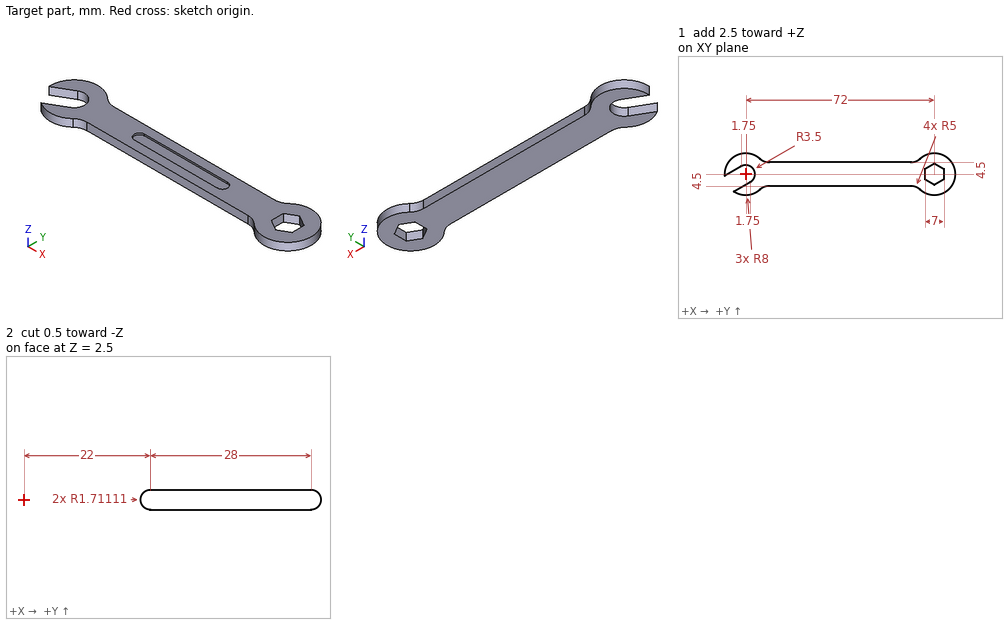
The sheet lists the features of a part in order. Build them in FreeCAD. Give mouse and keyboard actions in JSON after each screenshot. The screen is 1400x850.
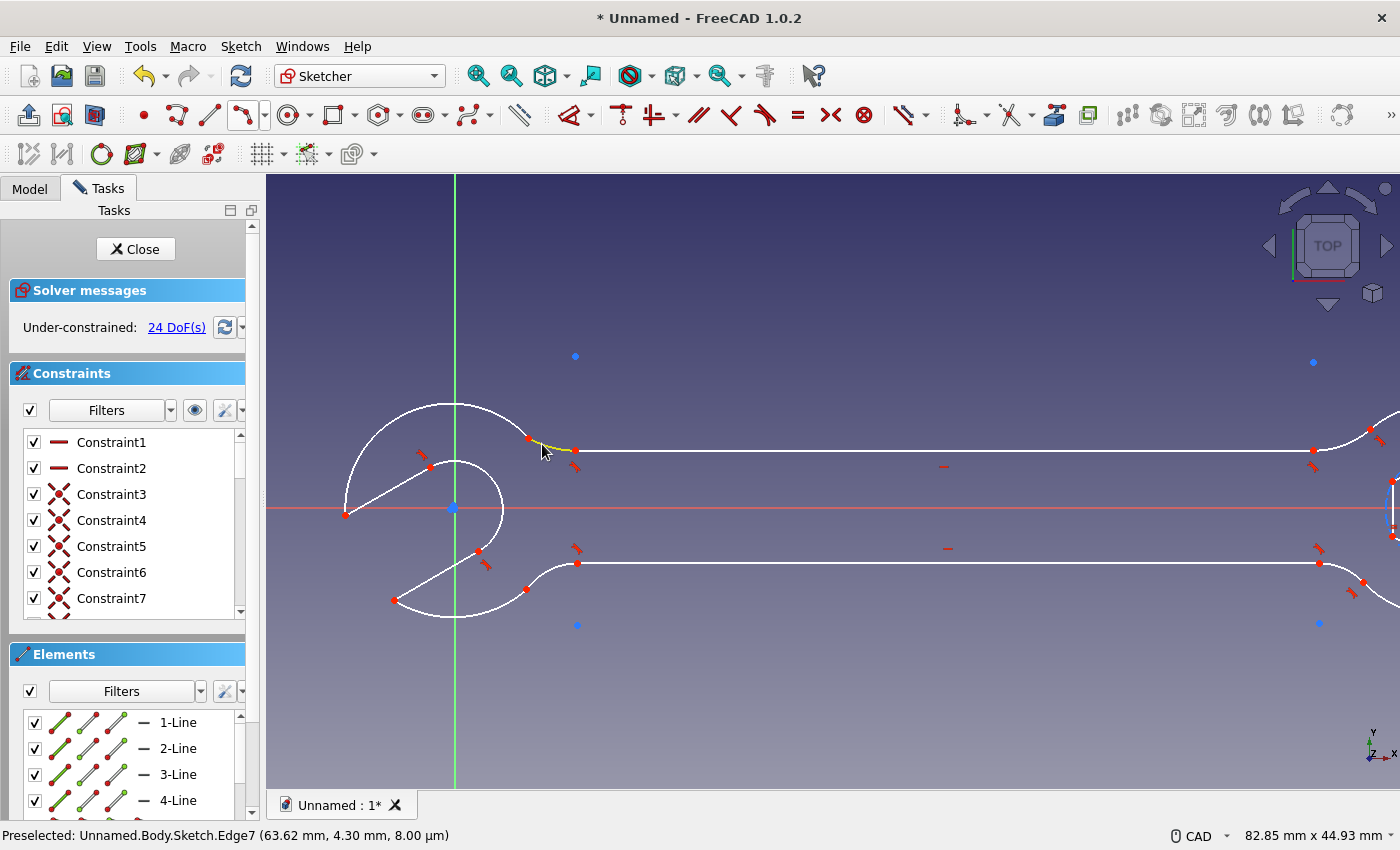
{"action": "left_click", "coordinate": [542, 444]}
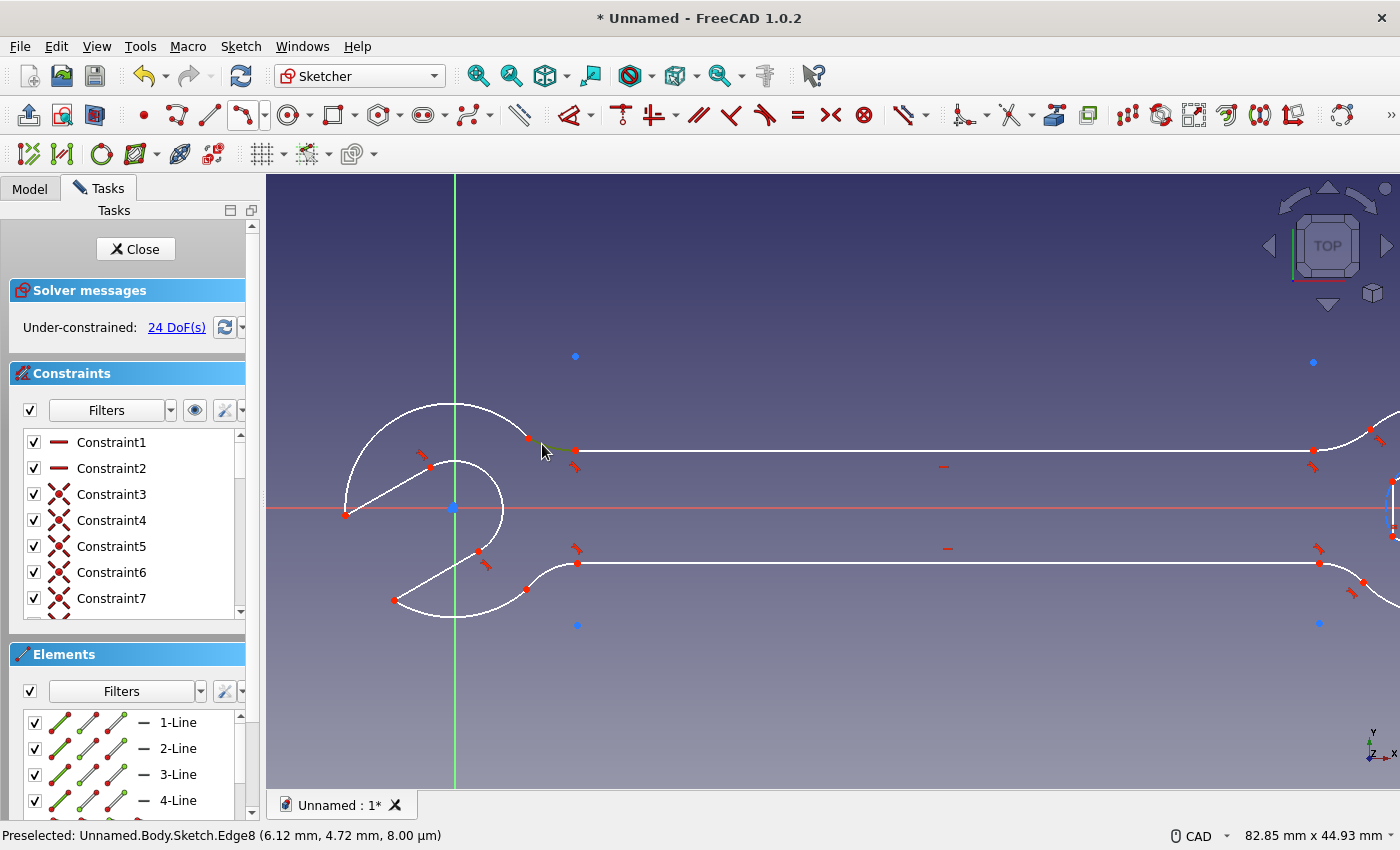
{"action": "left_click", "coordinate": [368, 443]}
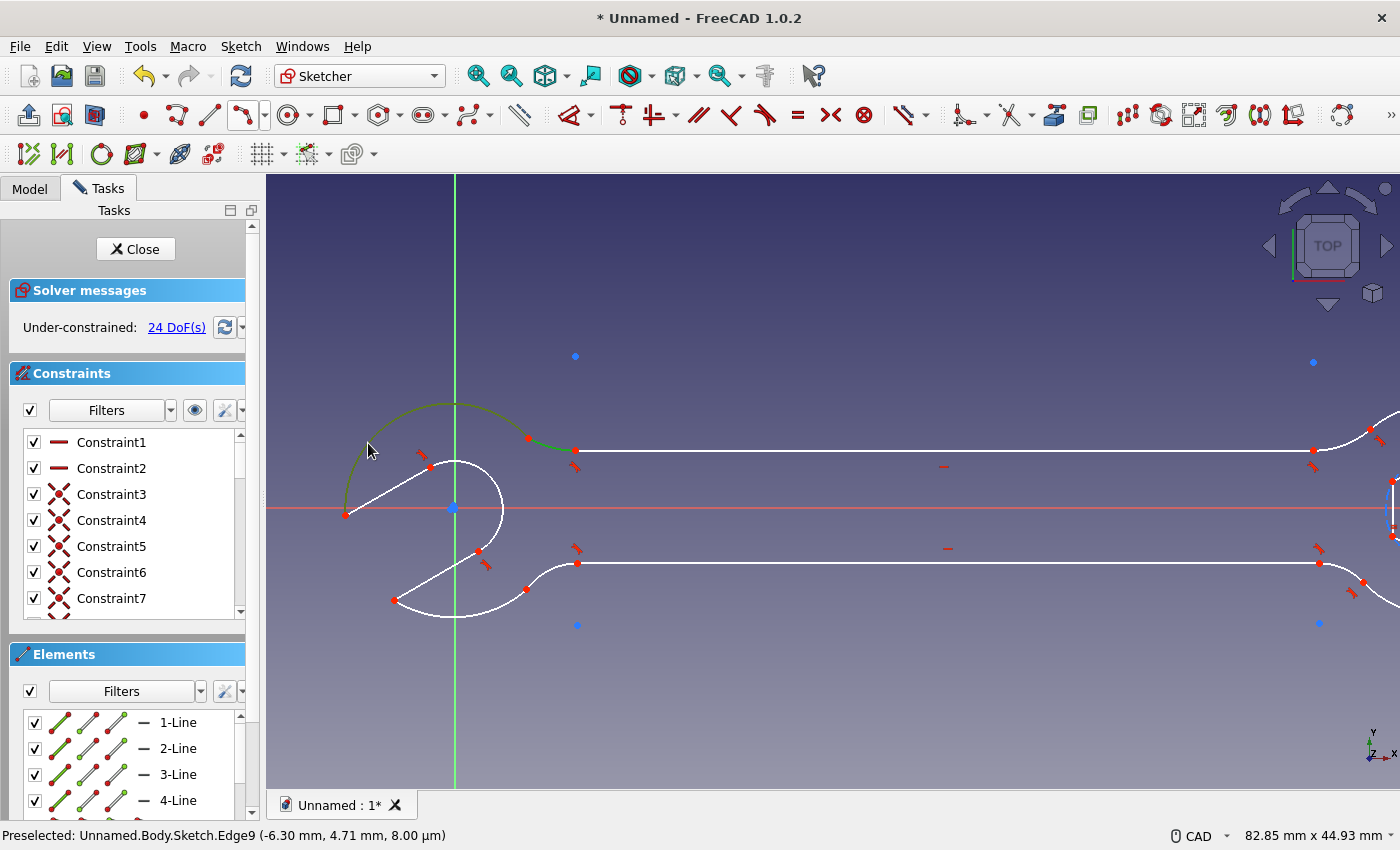
{"action": "key", "text": "t"}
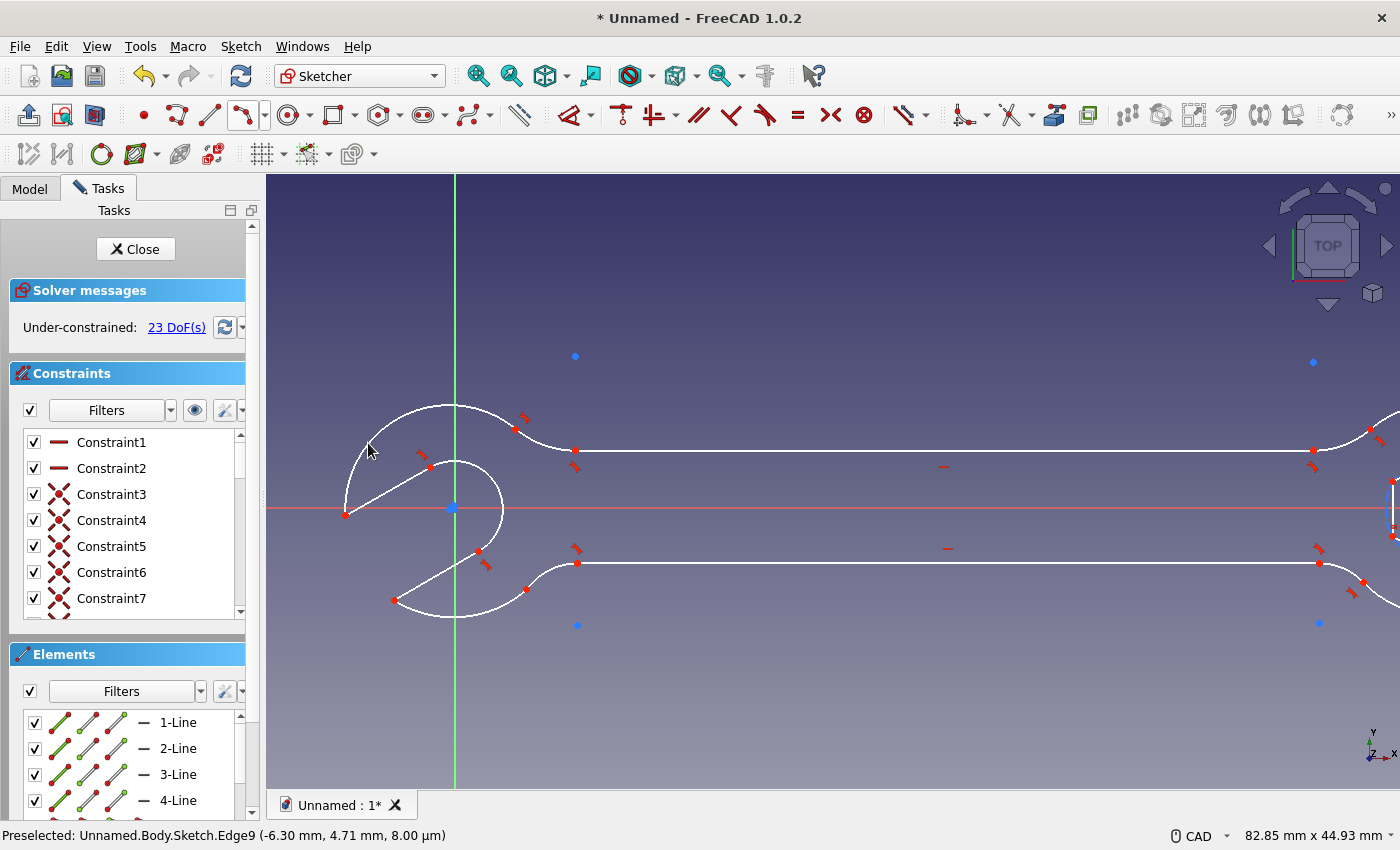
{"action": "left_click", "coordinate": [434, 616]}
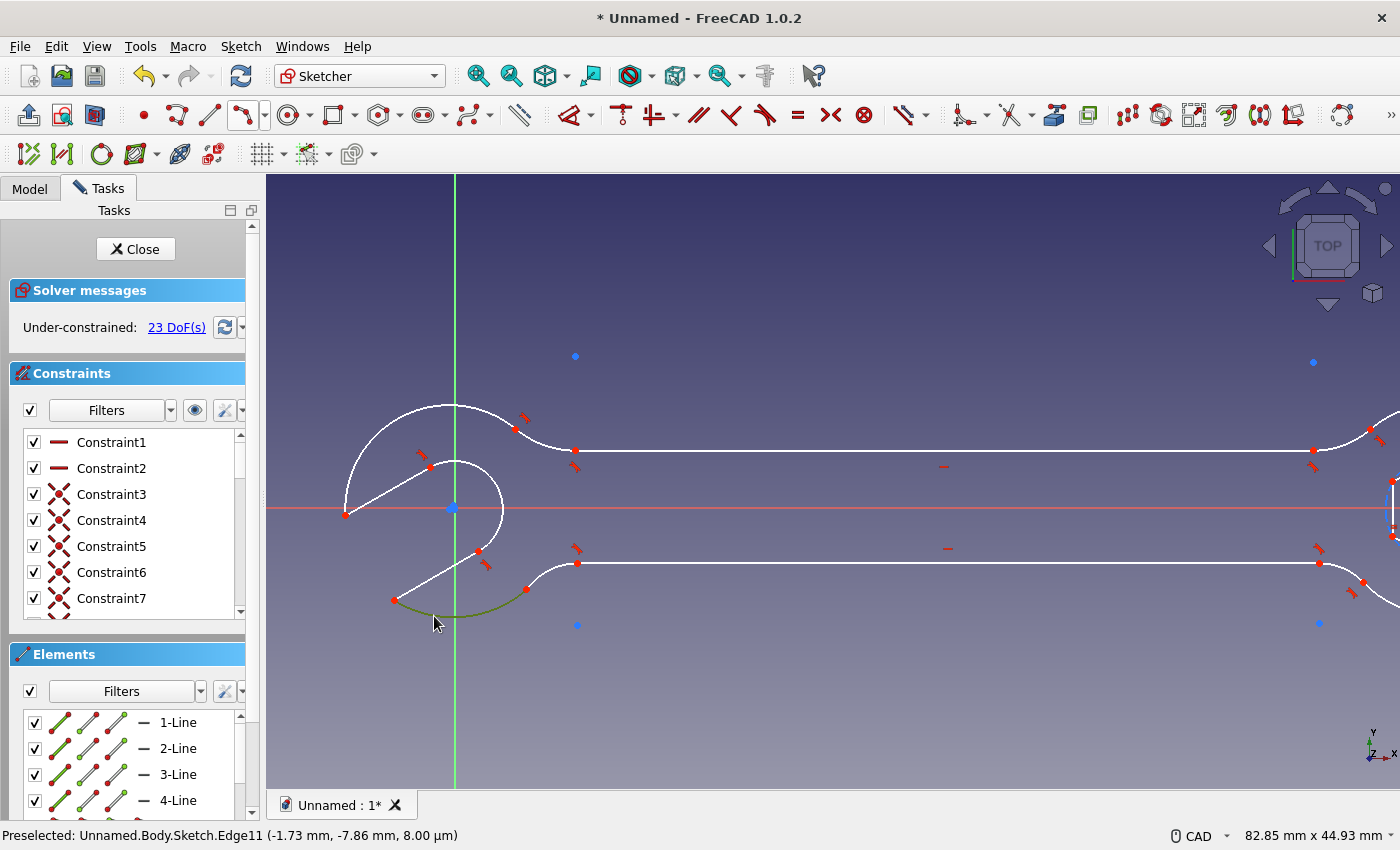
{"action": "left_click", "coordinate": [560, 566]}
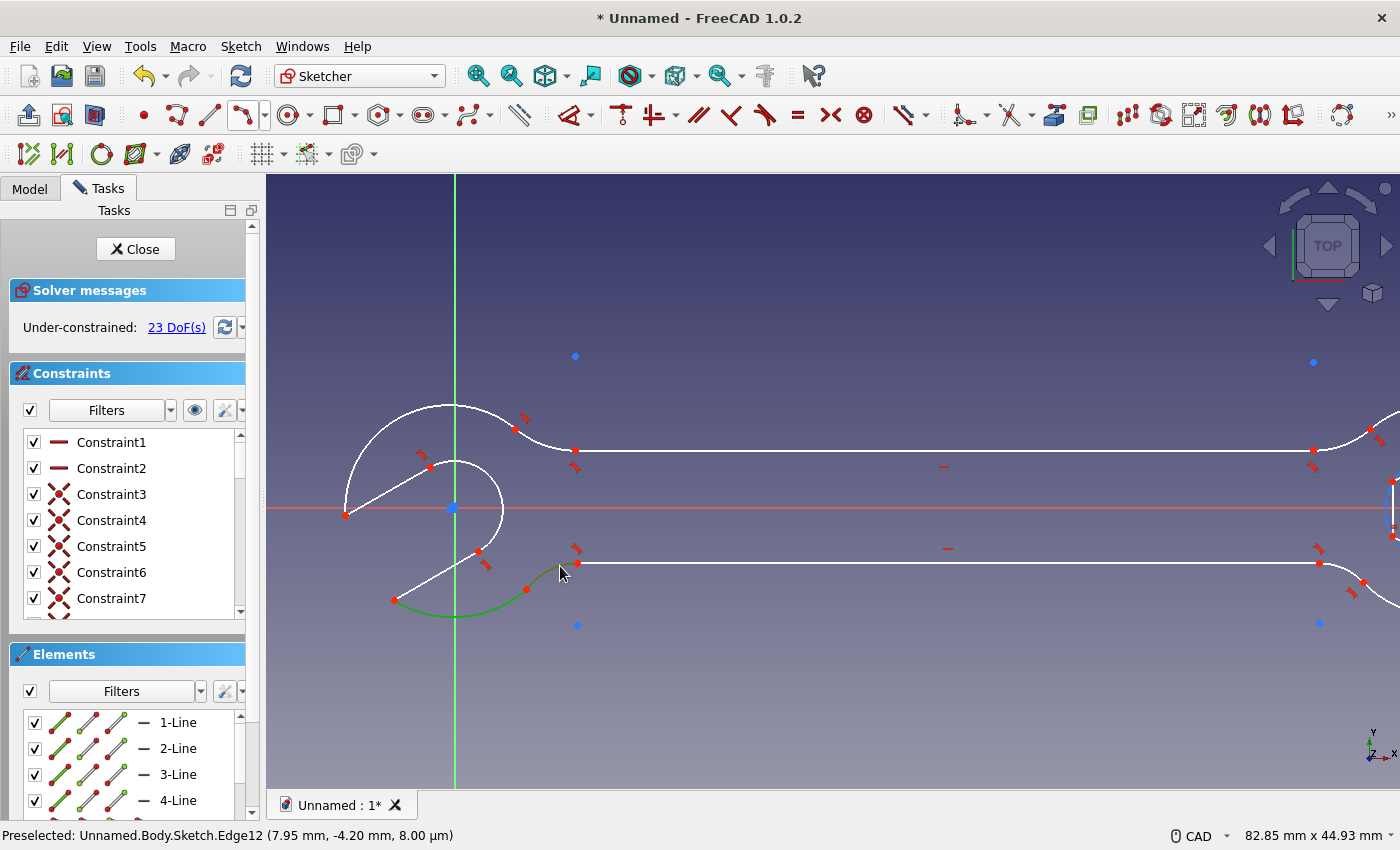
{"action": "left_click", "coordinate": [765, 116]}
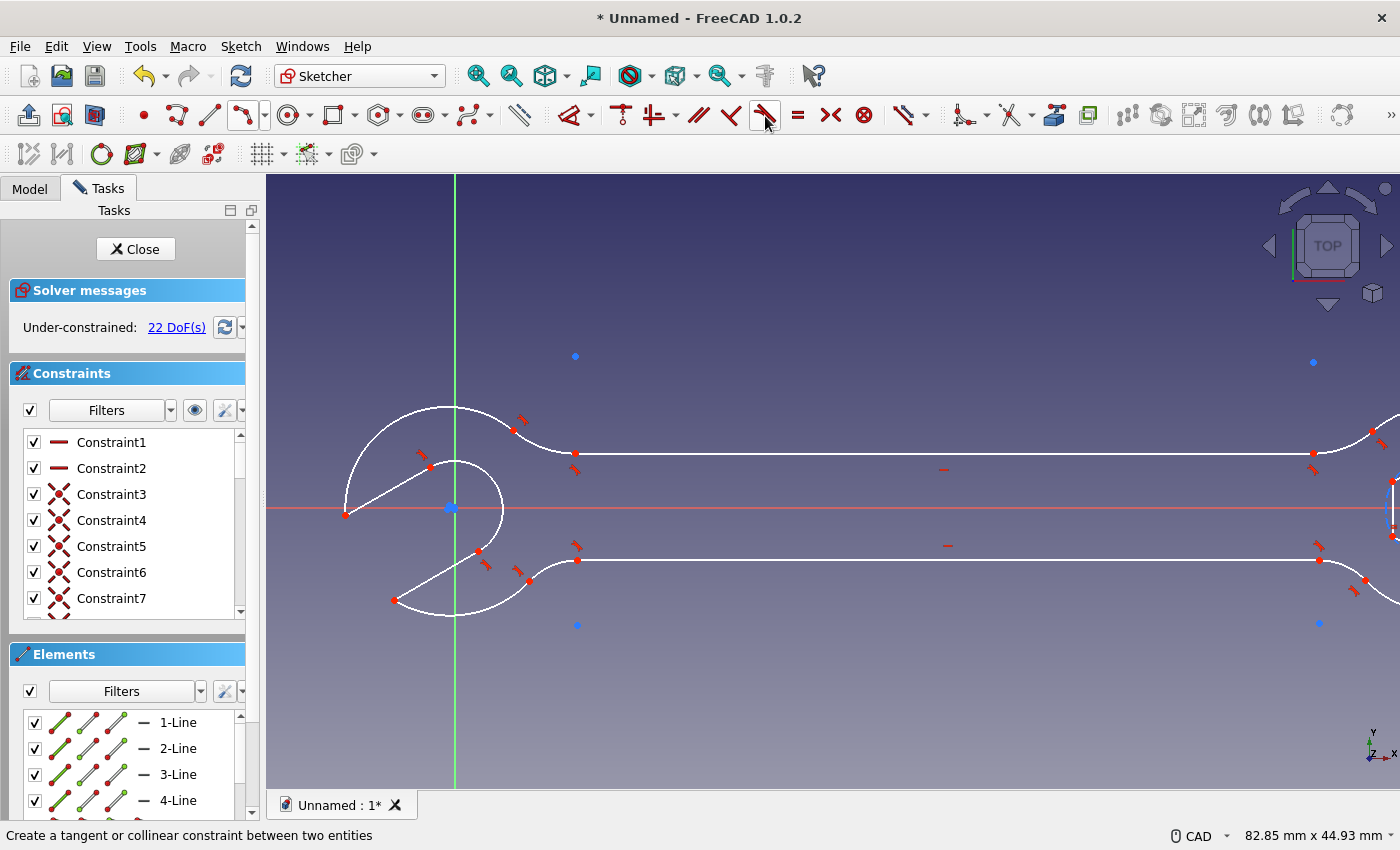
{"action": "scroll", "coordinate": [542, 444], "scroll_direction": "down", "scroll_amount": 3}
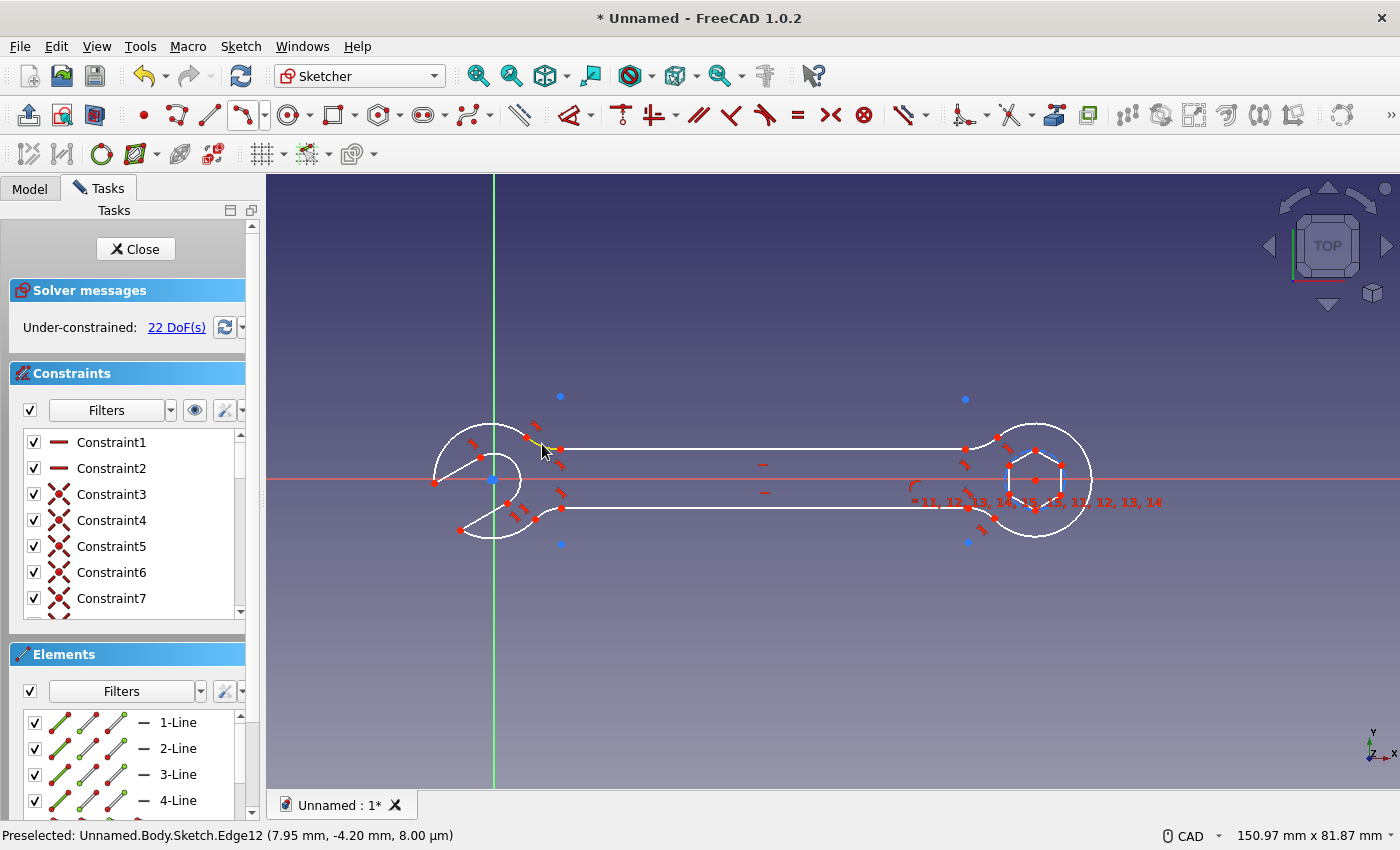
{"action": "scroll", "coordinate": [1061, 480], "scroll_direction": "up", "scroll_amount": 7}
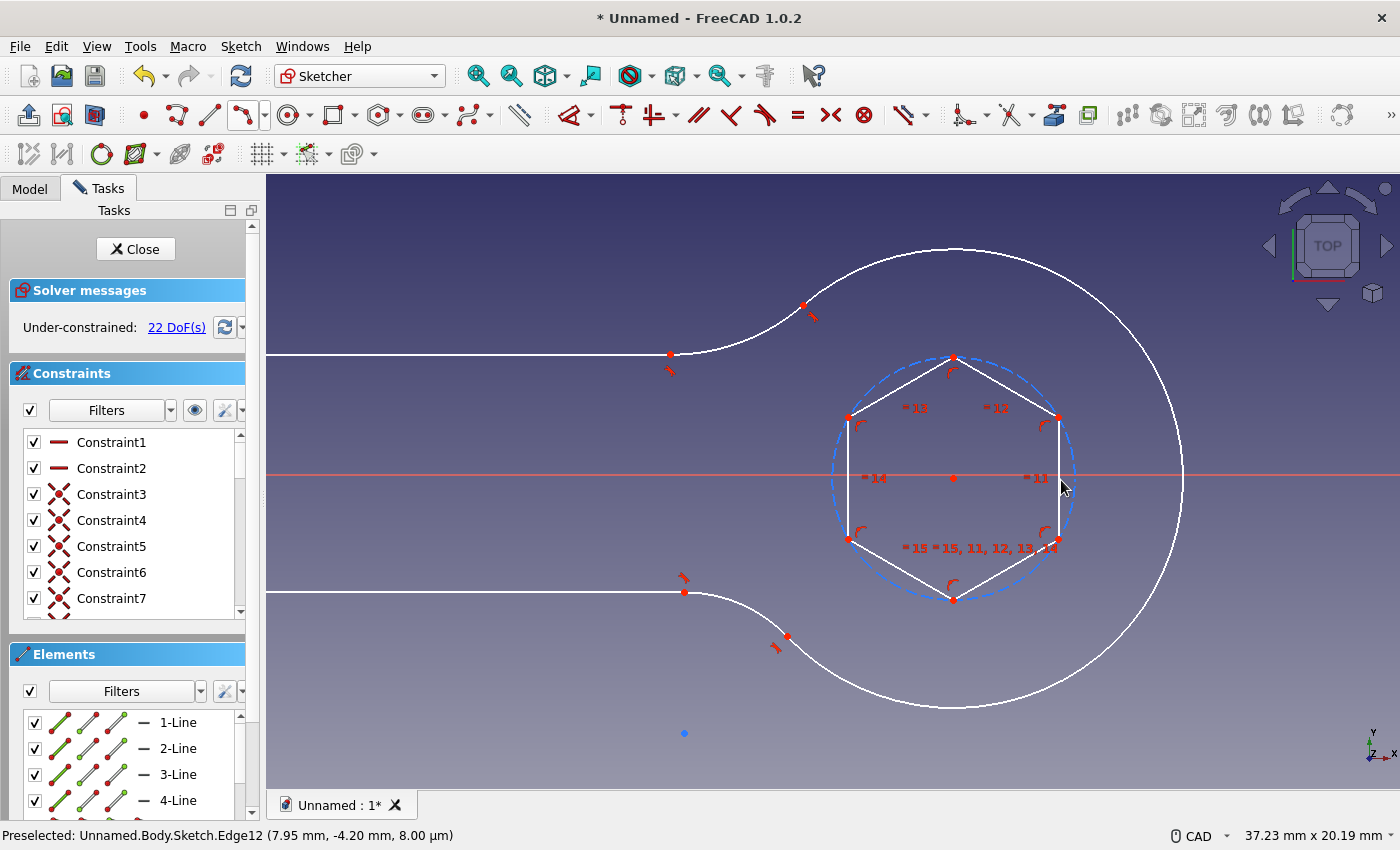
{"action": "left_click", "coordinate": [1059, 479]}